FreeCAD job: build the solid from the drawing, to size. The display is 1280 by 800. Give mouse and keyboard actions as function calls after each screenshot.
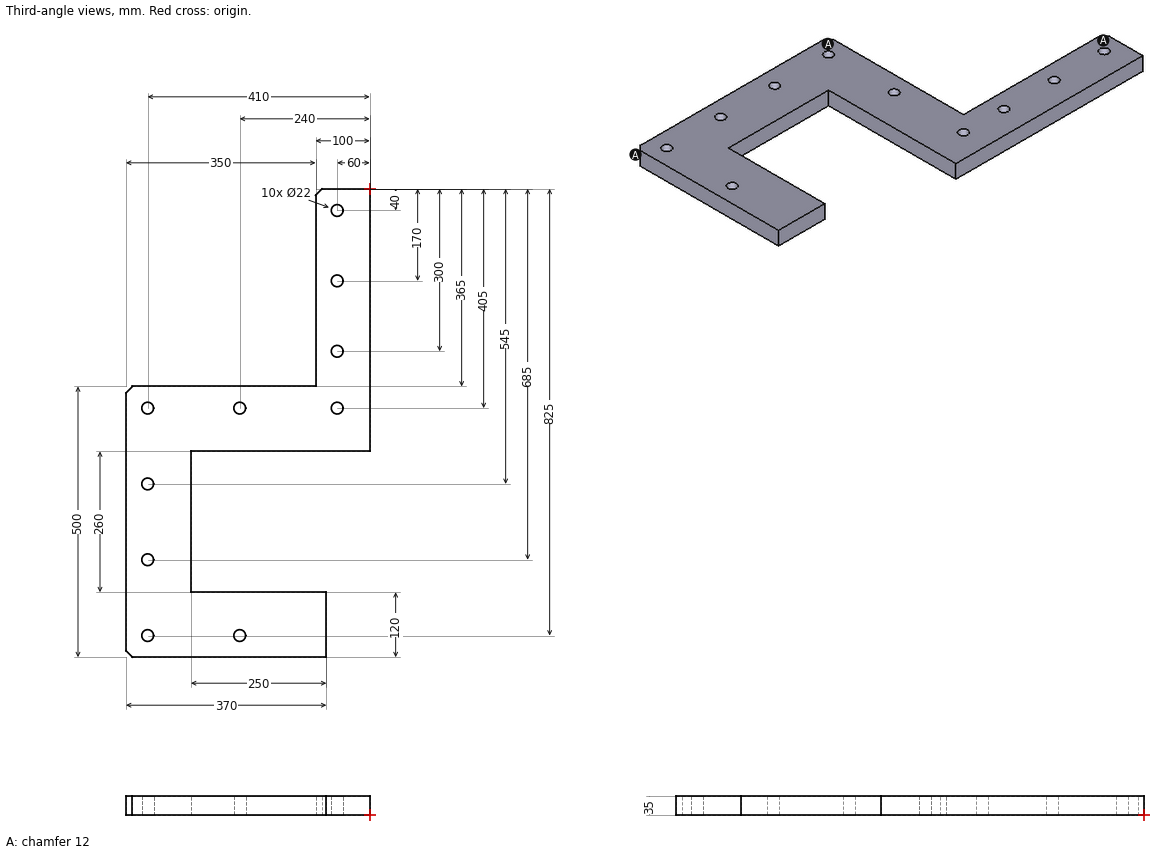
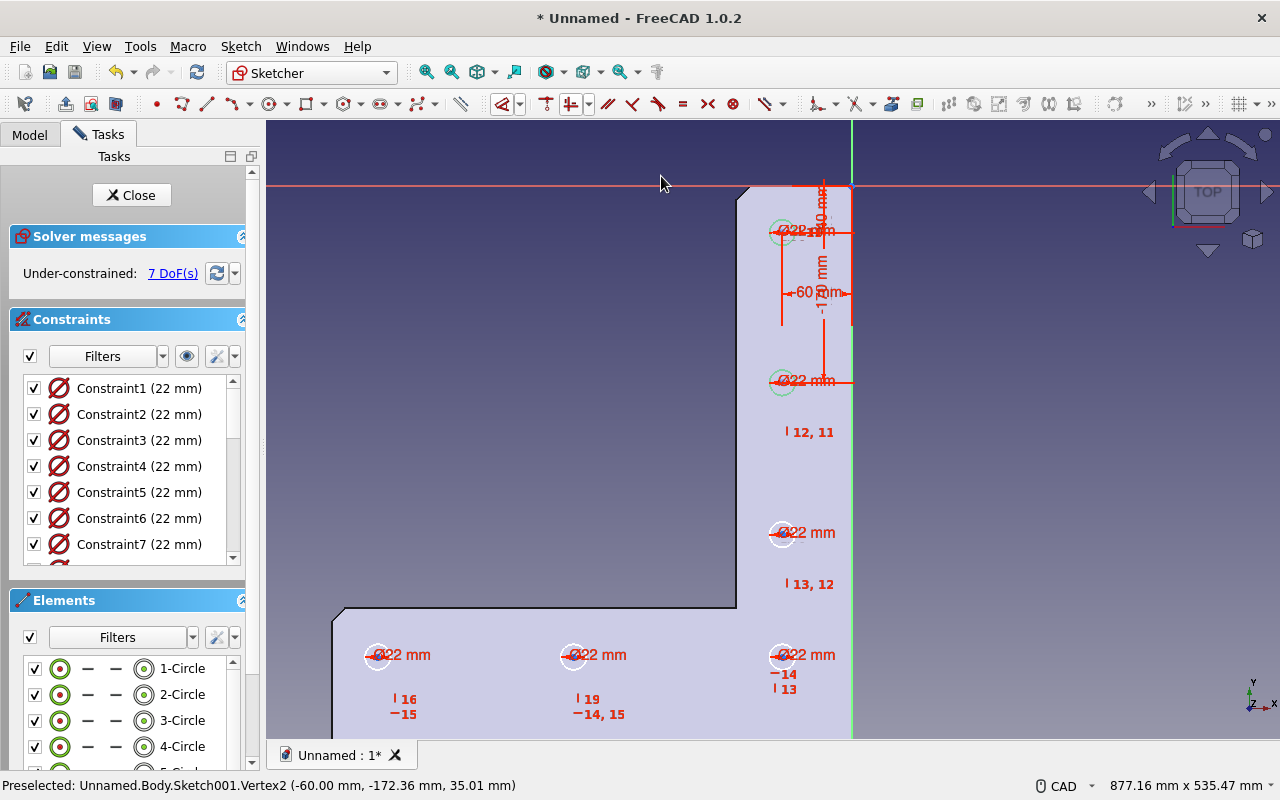
click(782, 535)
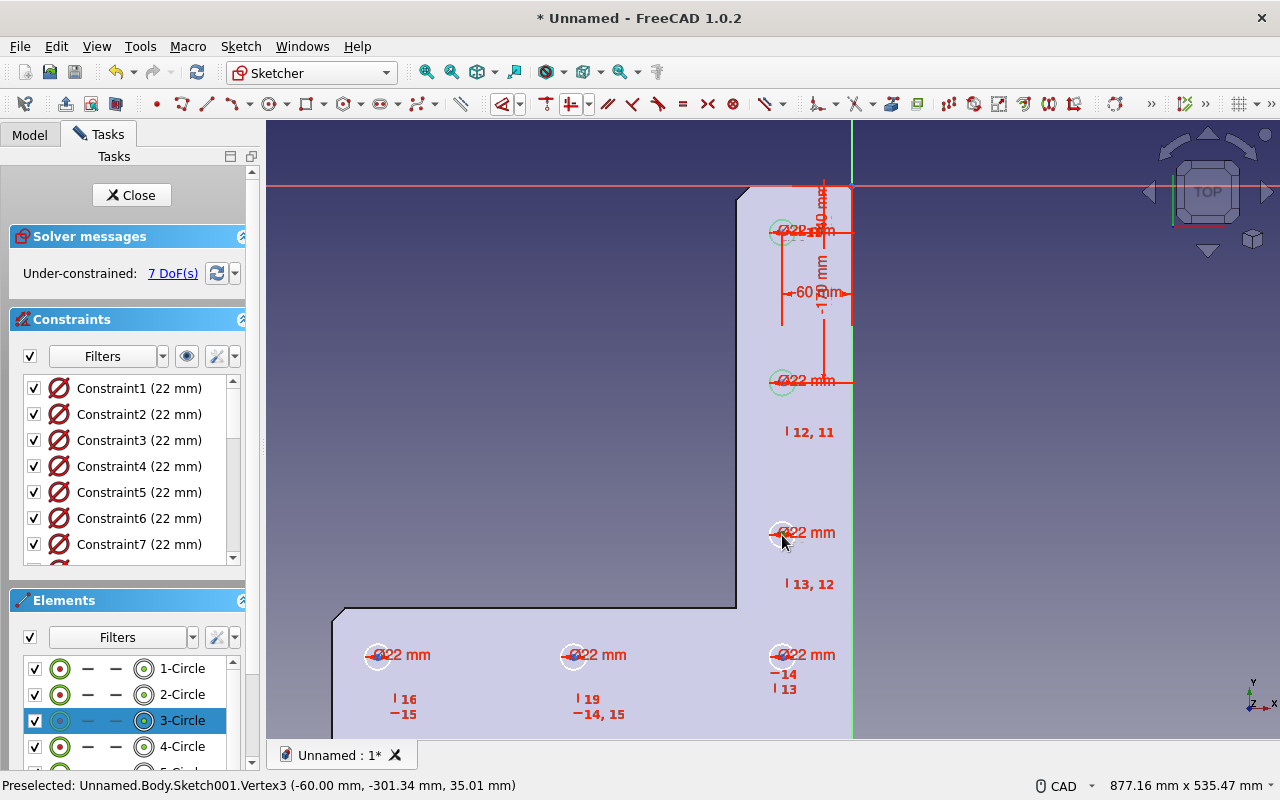
click(520, 104)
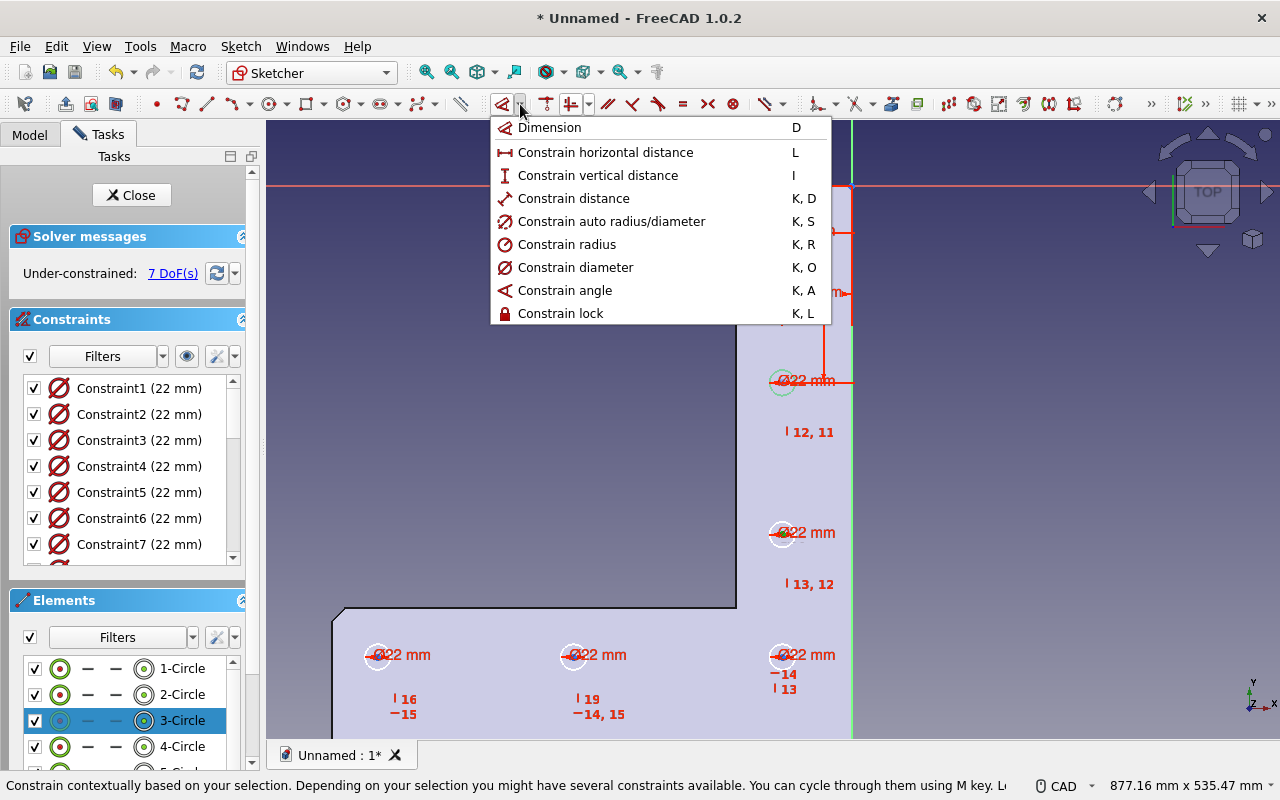
click(661, 176)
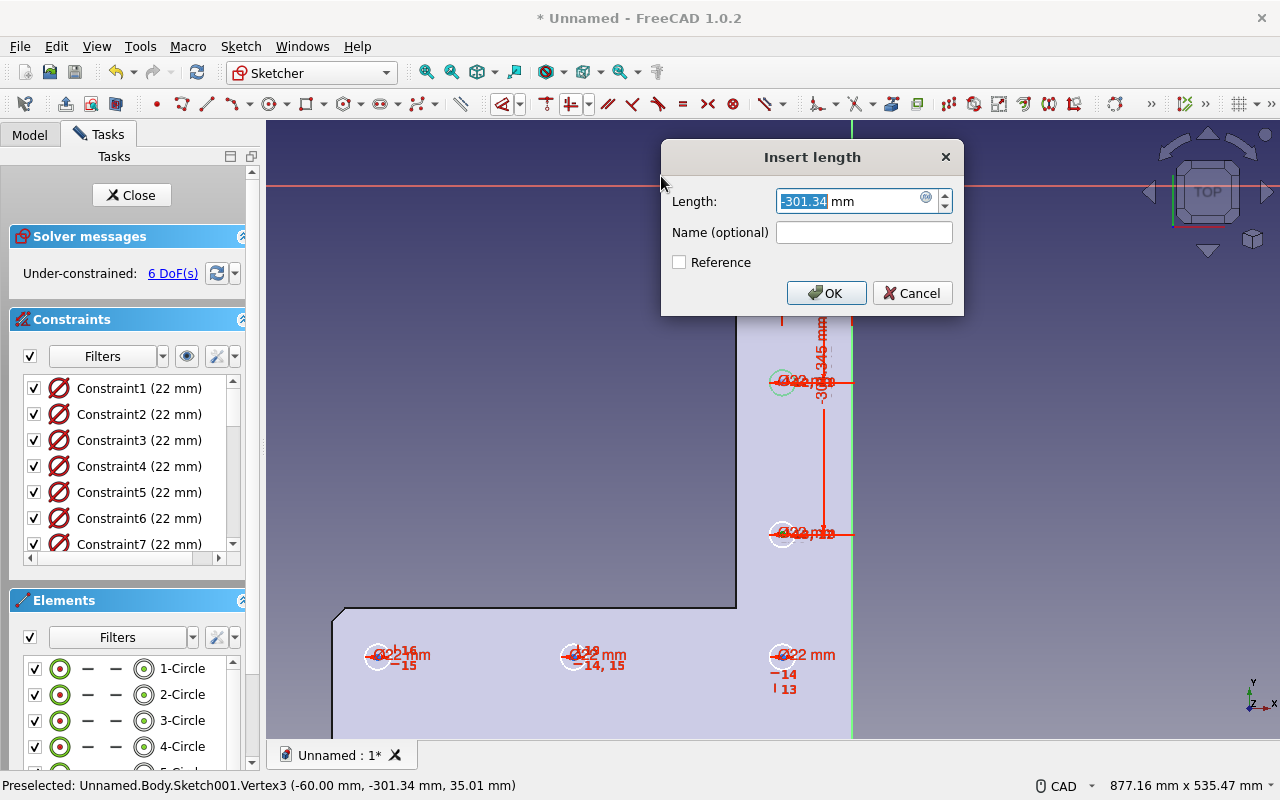
text(-300)
key(Return)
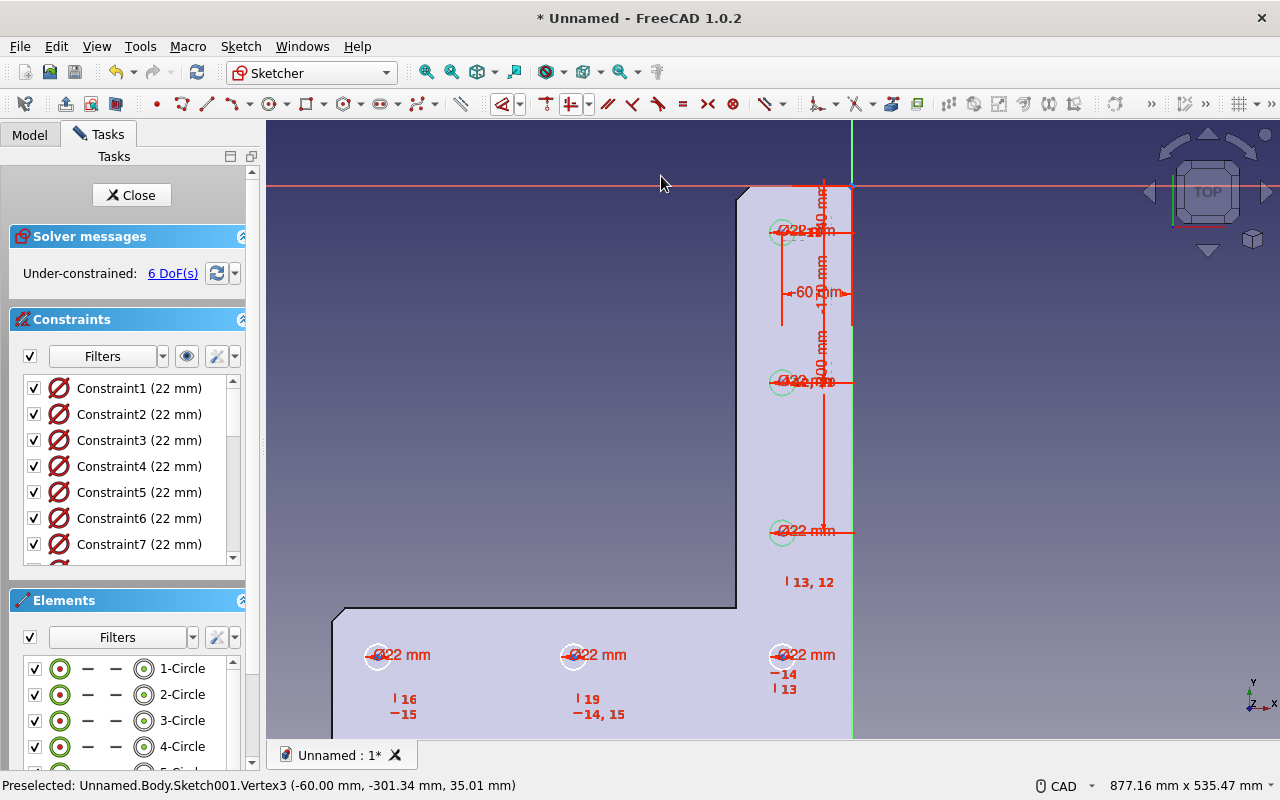
click(782, 657)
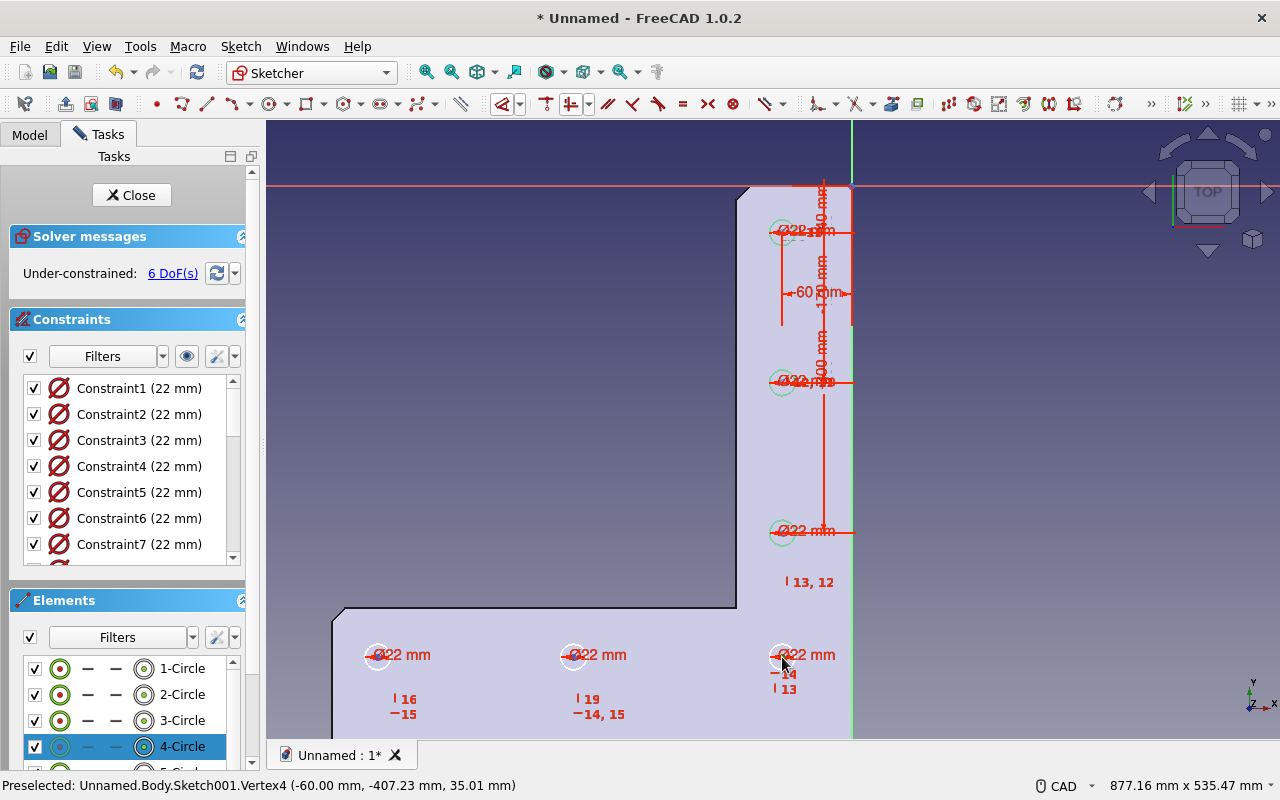
click(520, 104)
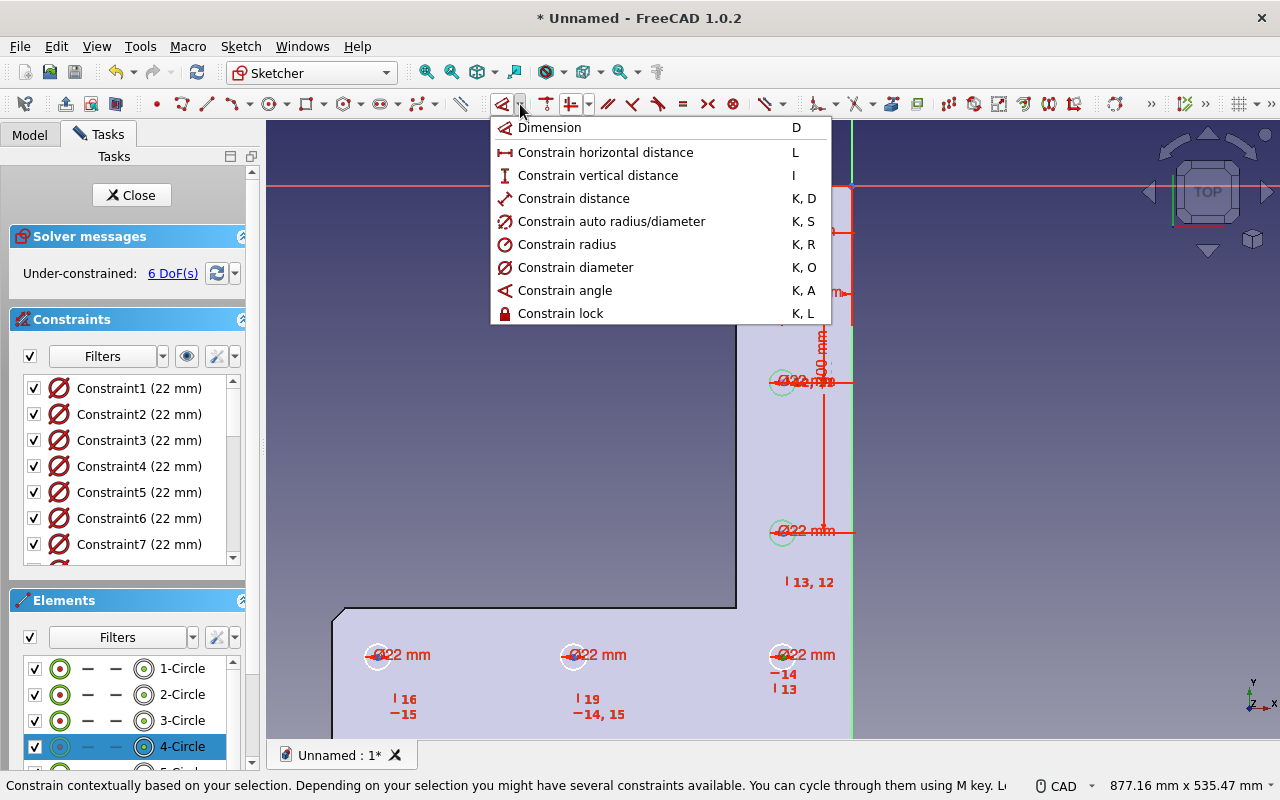
click(661, 176)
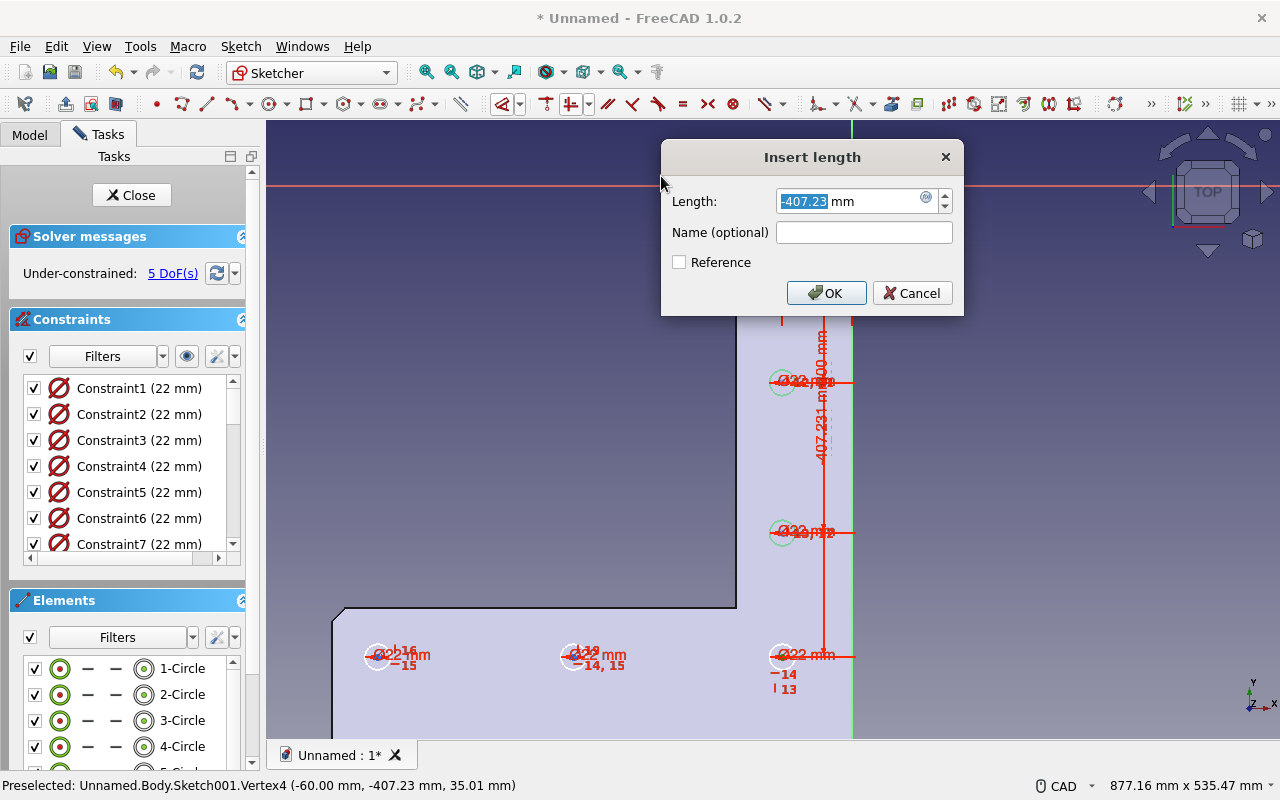
text(-405)
key(Return)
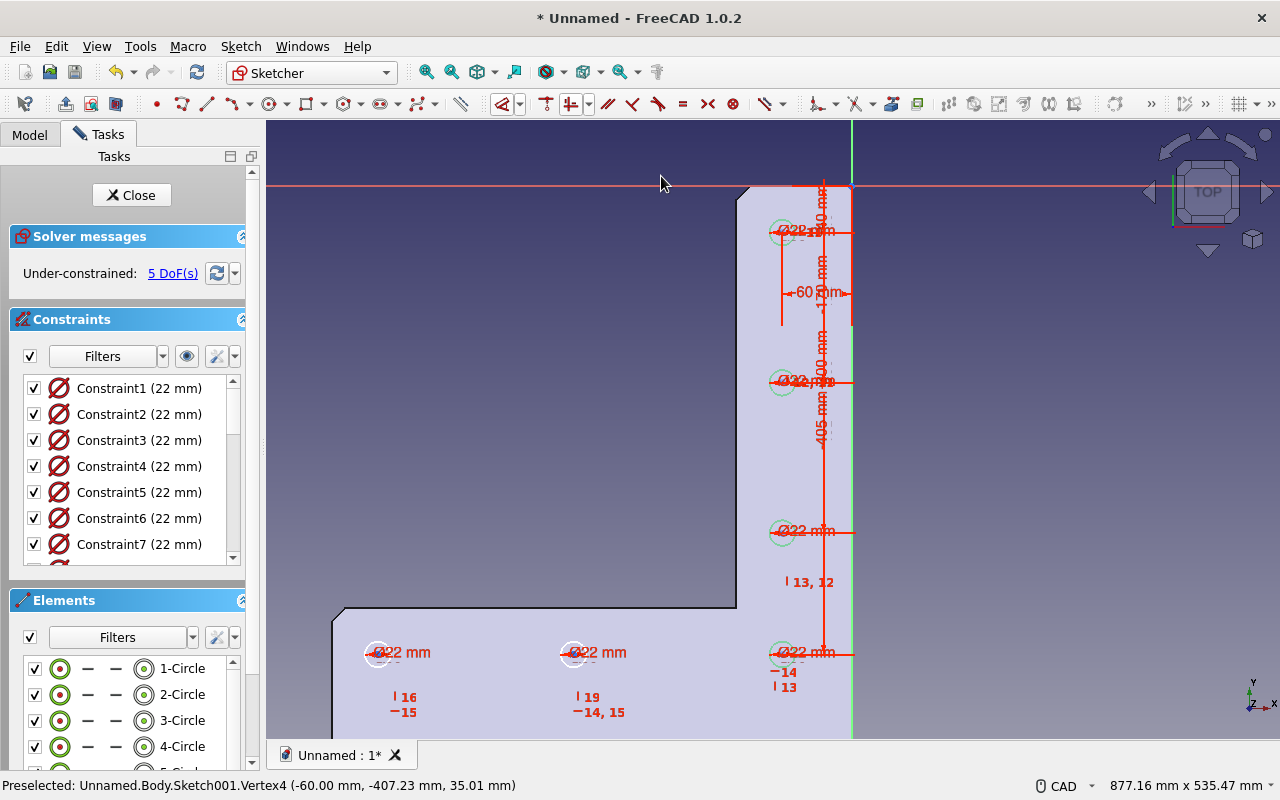
click(574, 654)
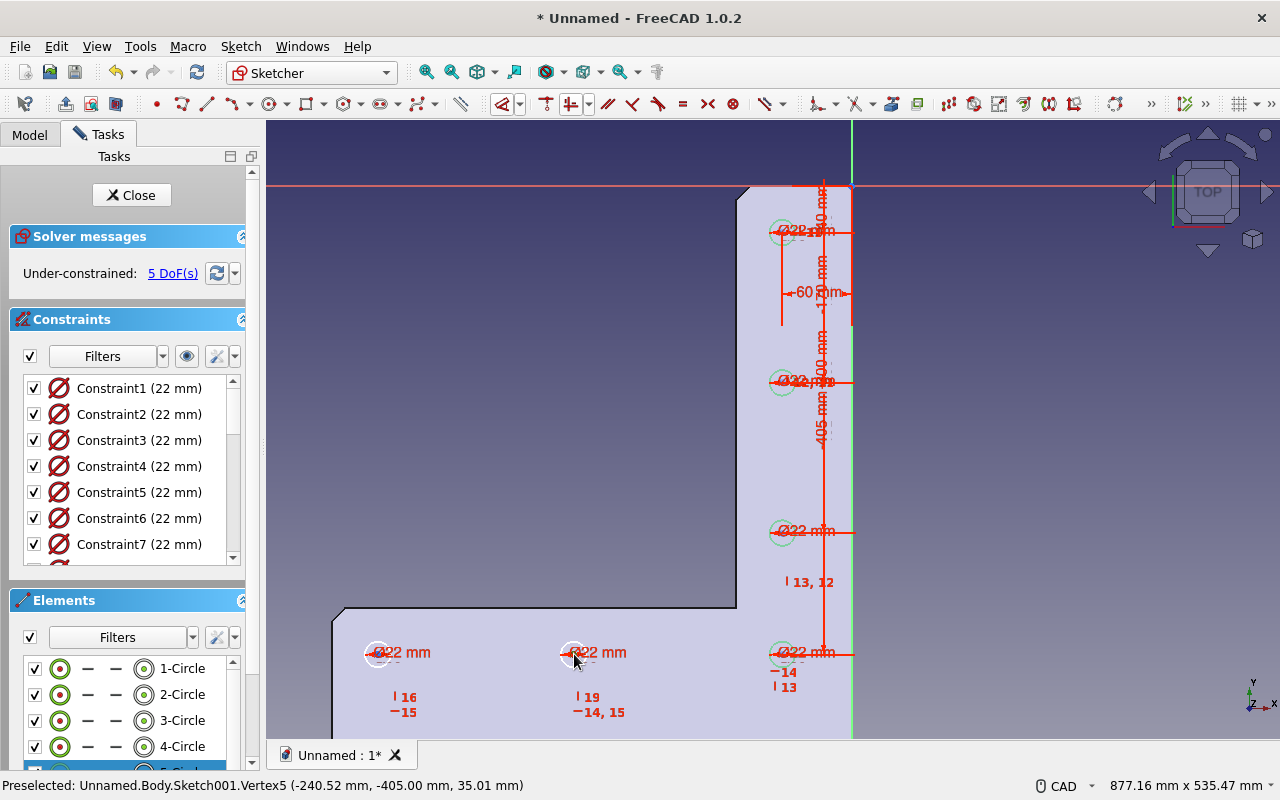
key(l)